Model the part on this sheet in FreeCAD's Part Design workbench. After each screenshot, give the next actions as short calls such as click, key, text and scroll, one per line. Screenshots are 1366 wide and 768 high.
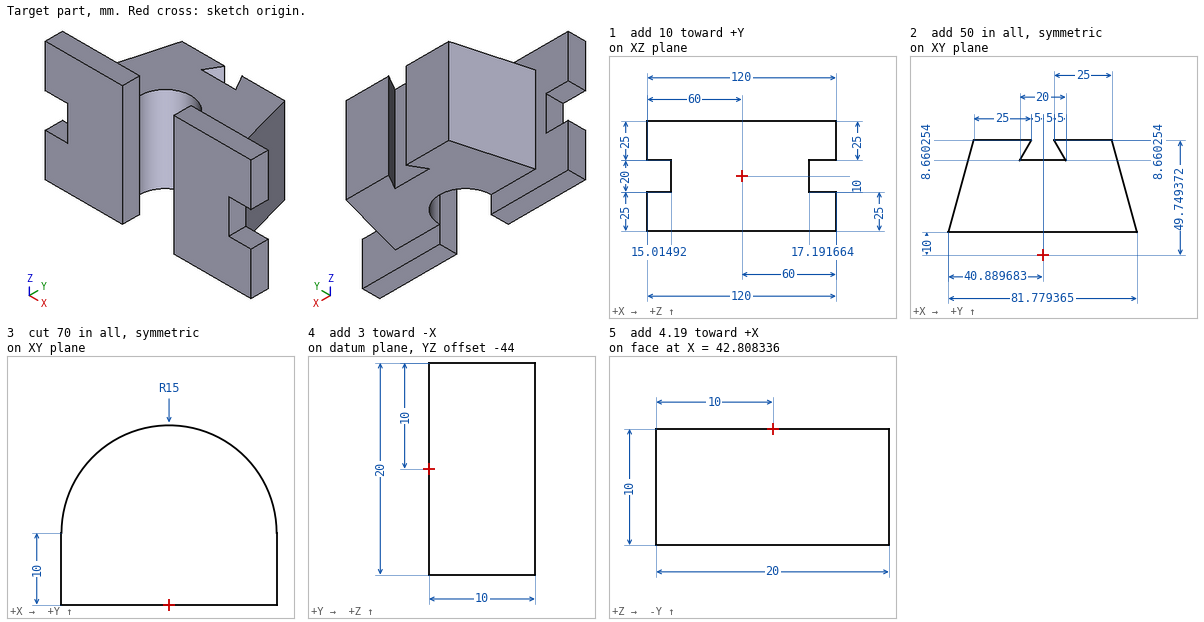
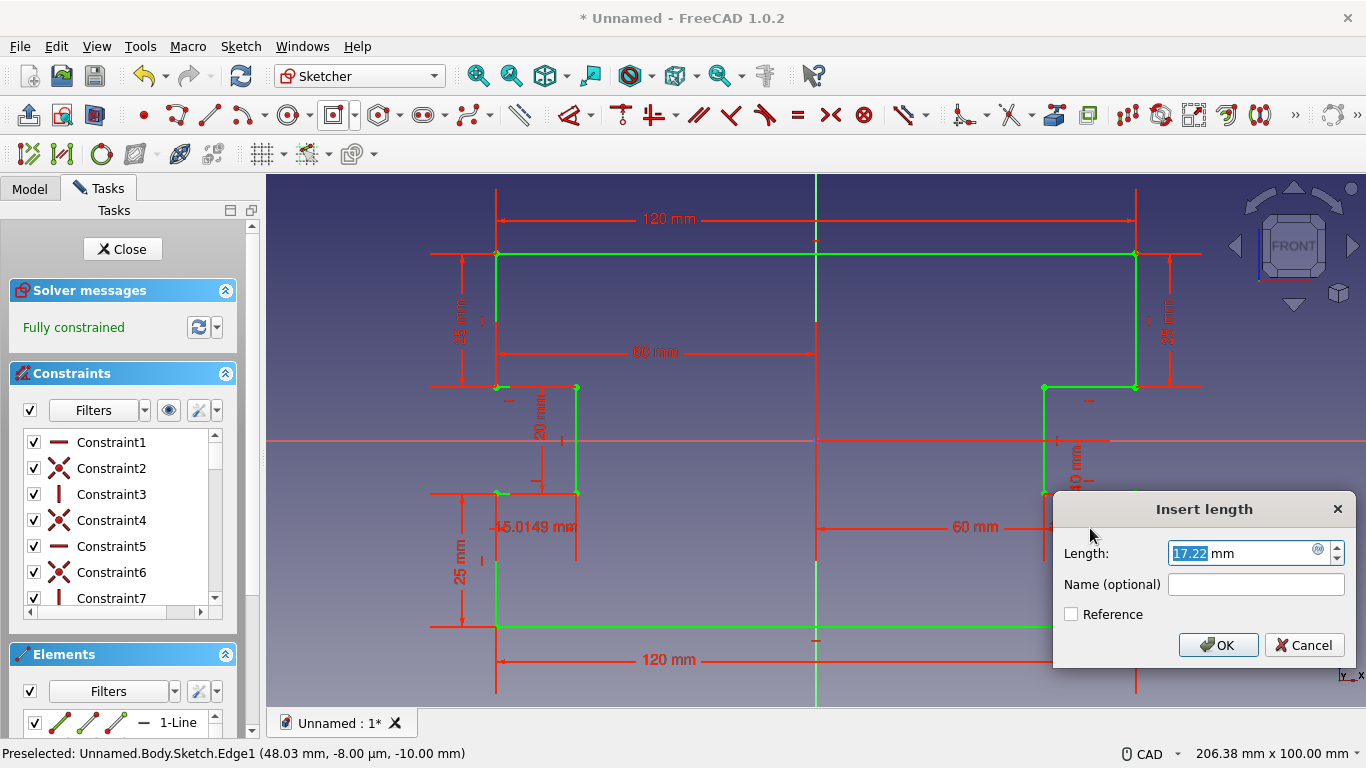
text(17.191664)
key(Return)
key(Escape)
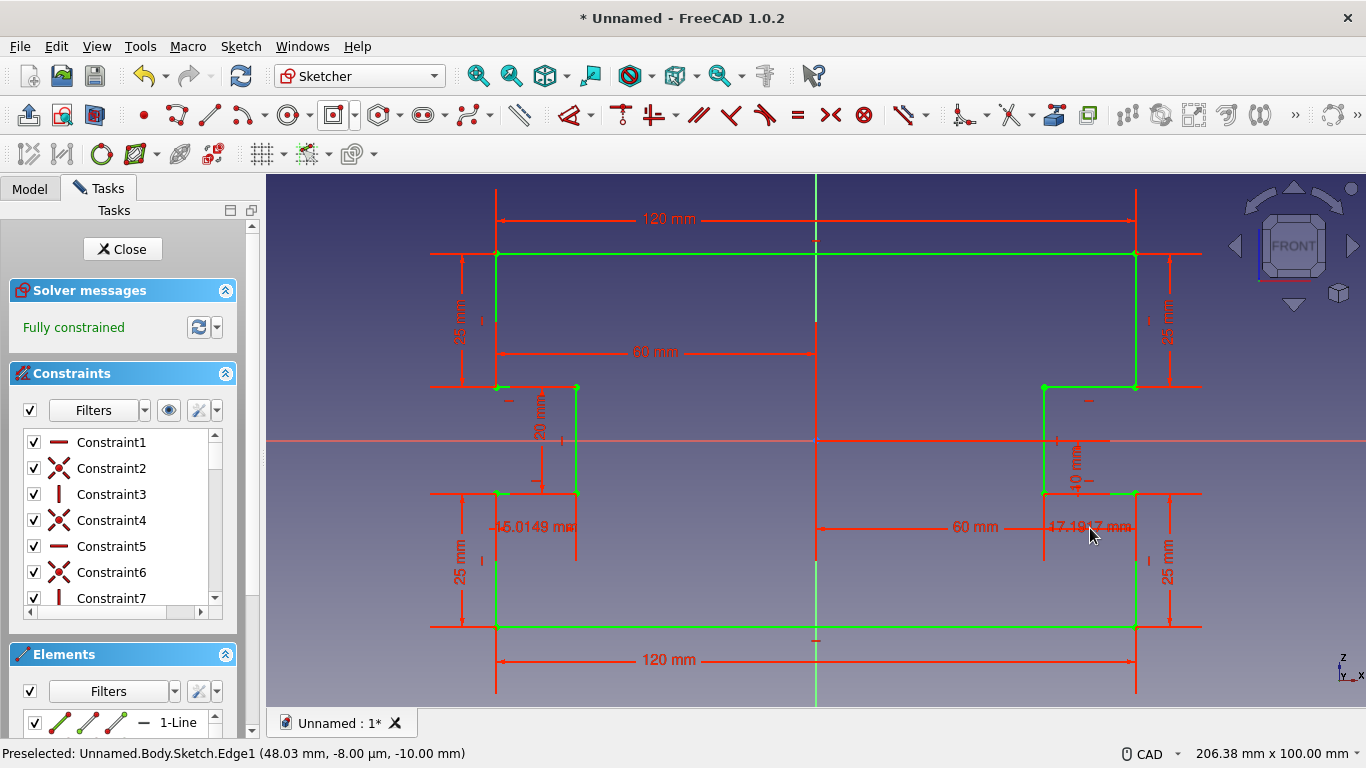
click(123, 249)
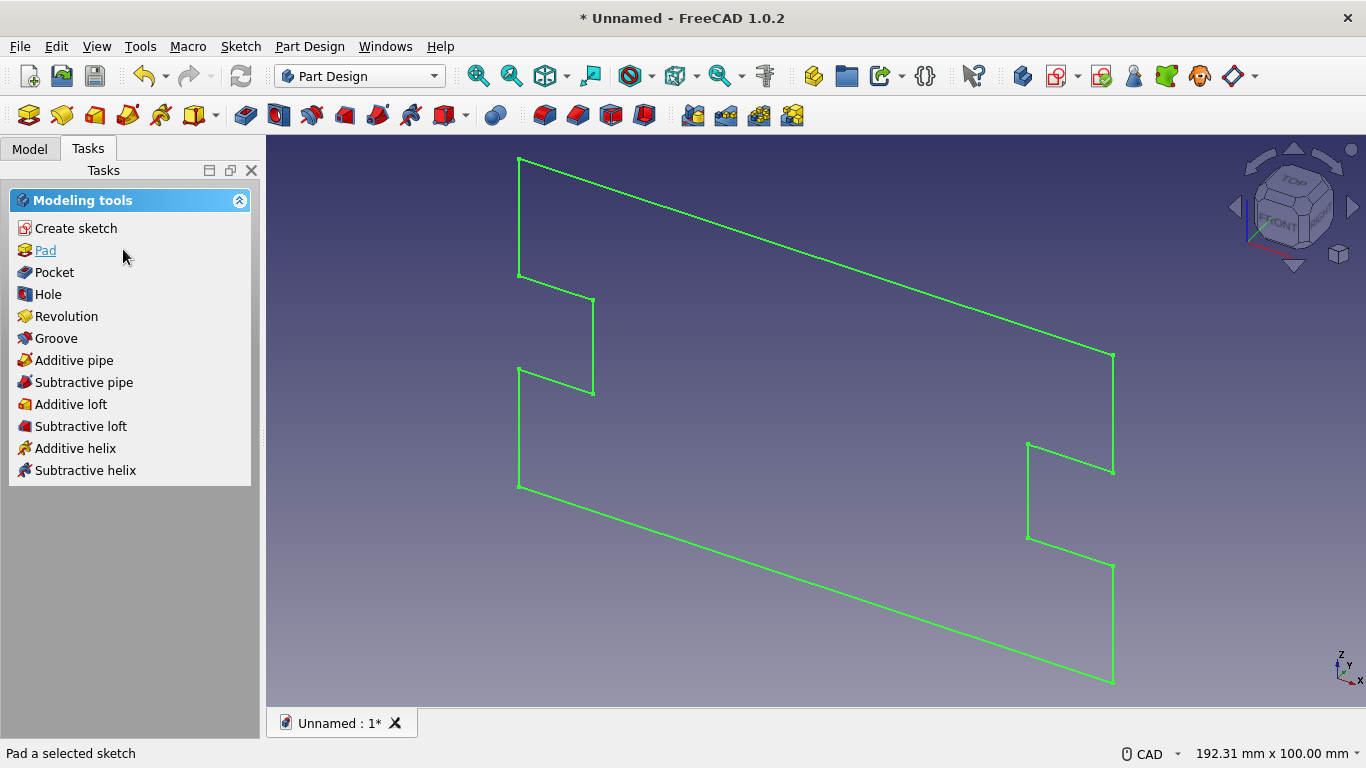
click(29, 116)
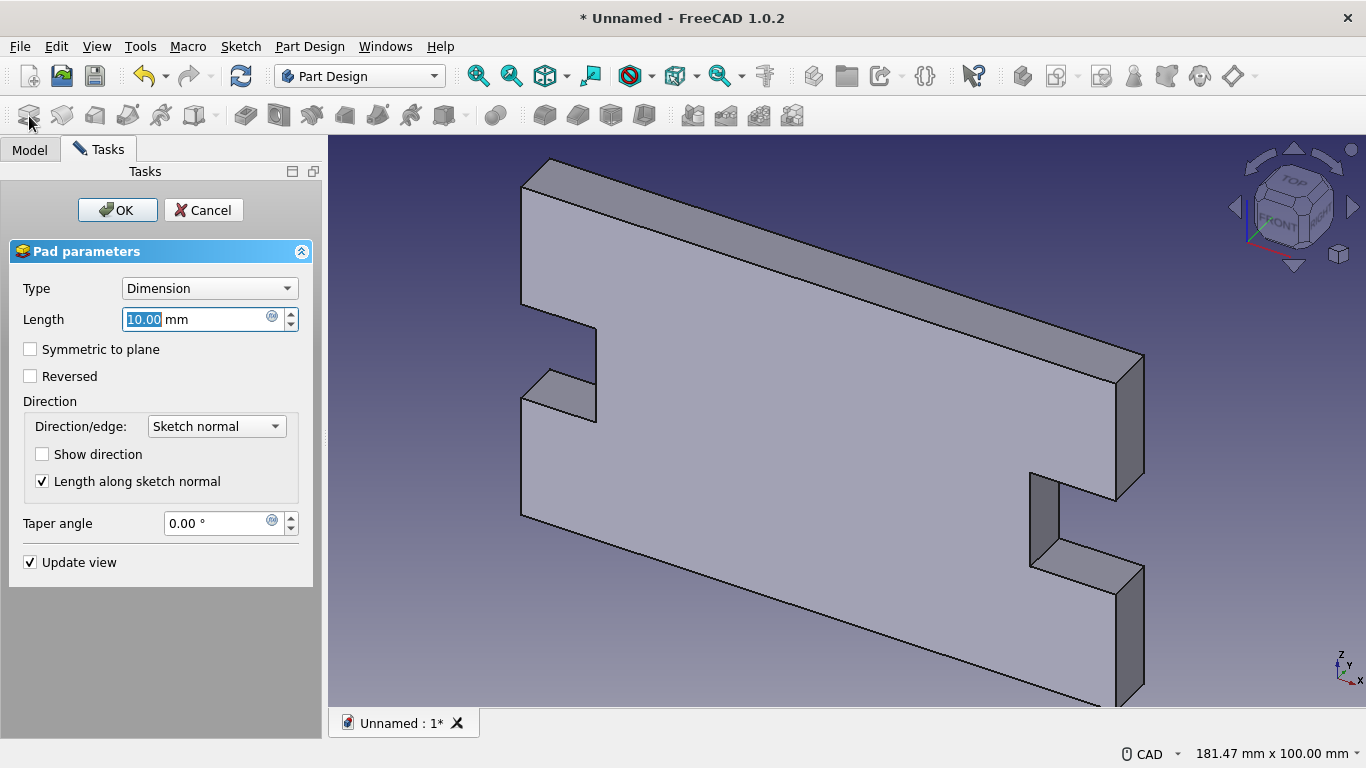
text(10)
key(Tab)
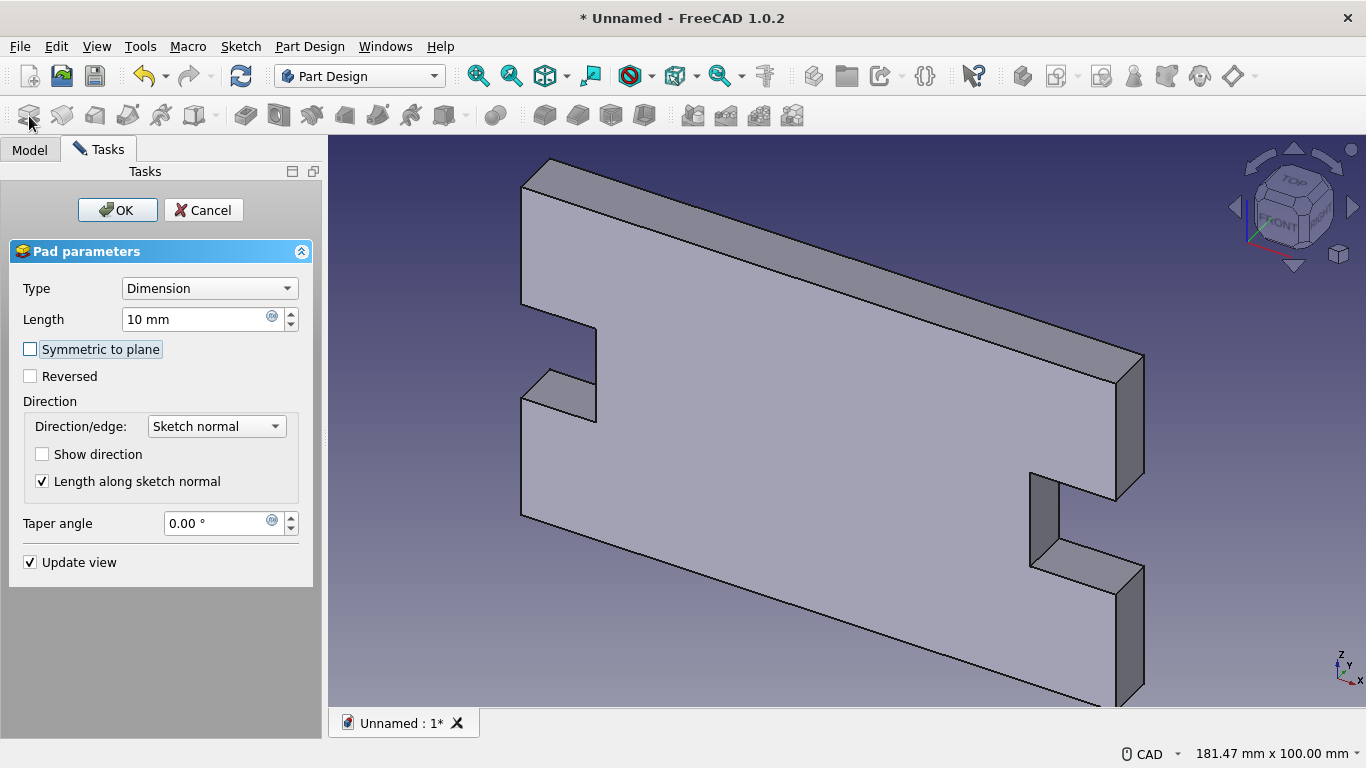
click(31, 376)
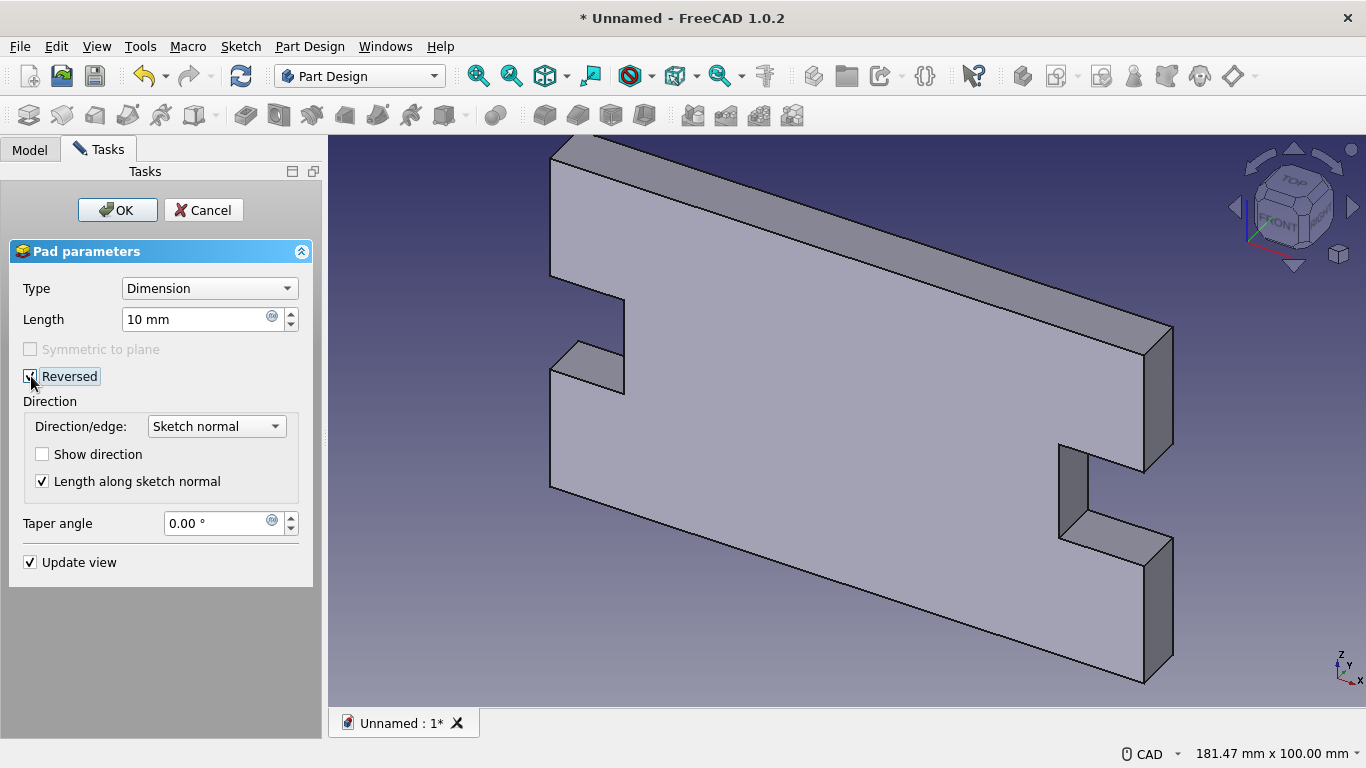
click(118, 210)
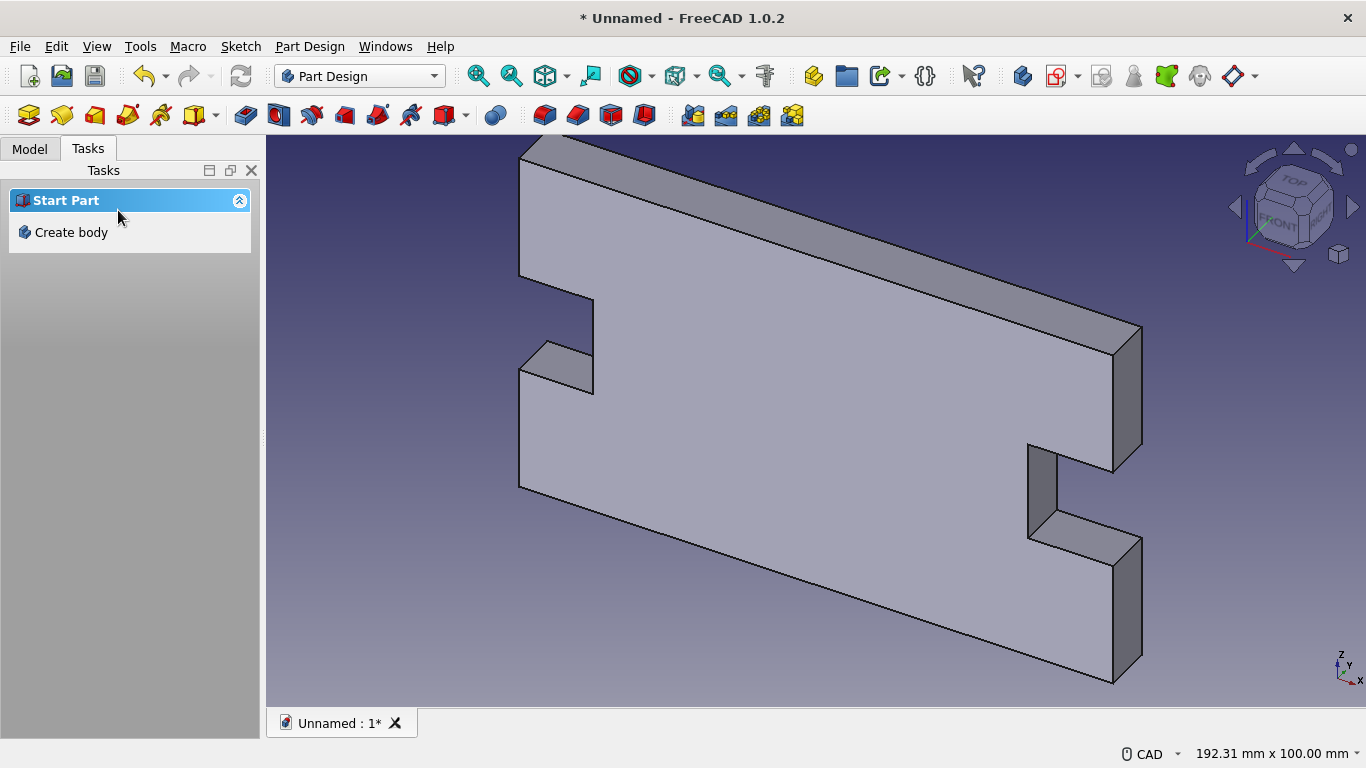
key(v)
key(f)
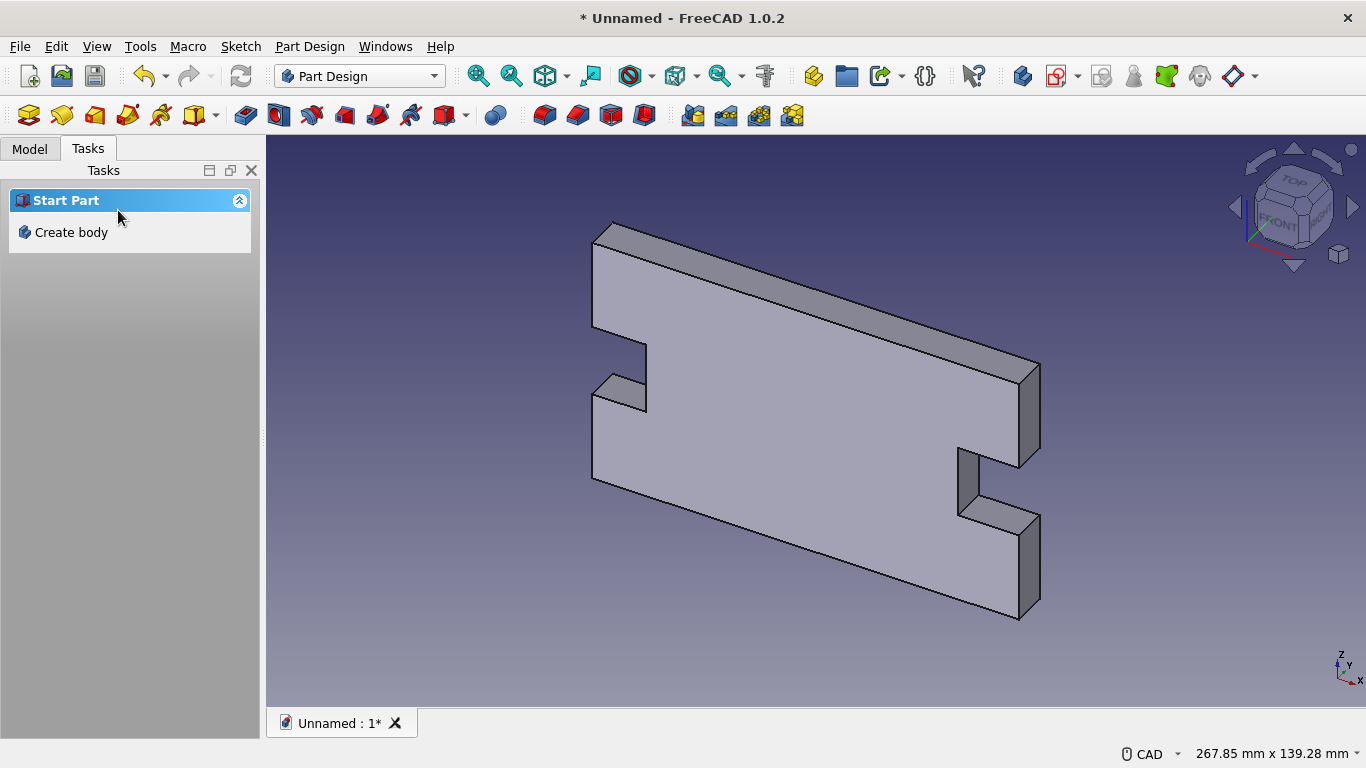
click(1056, 76)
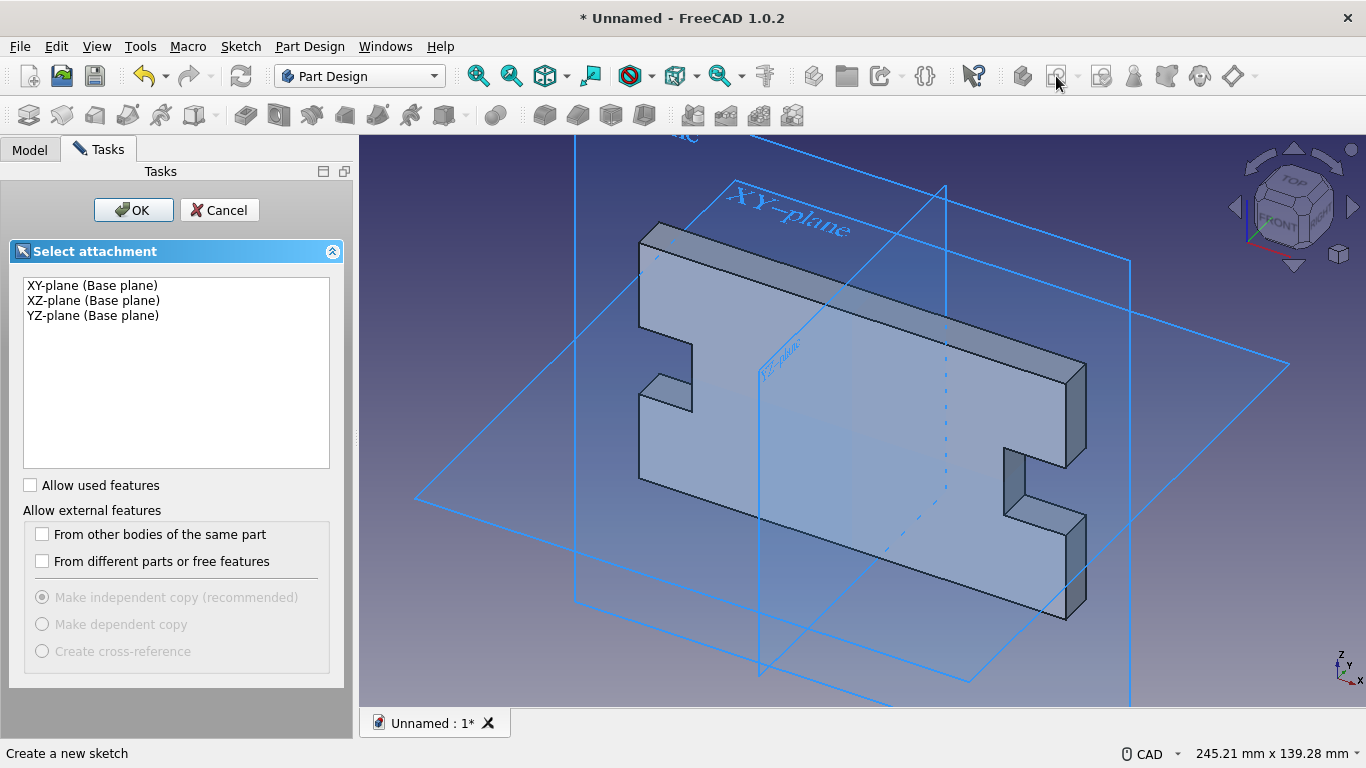
click(84, 286)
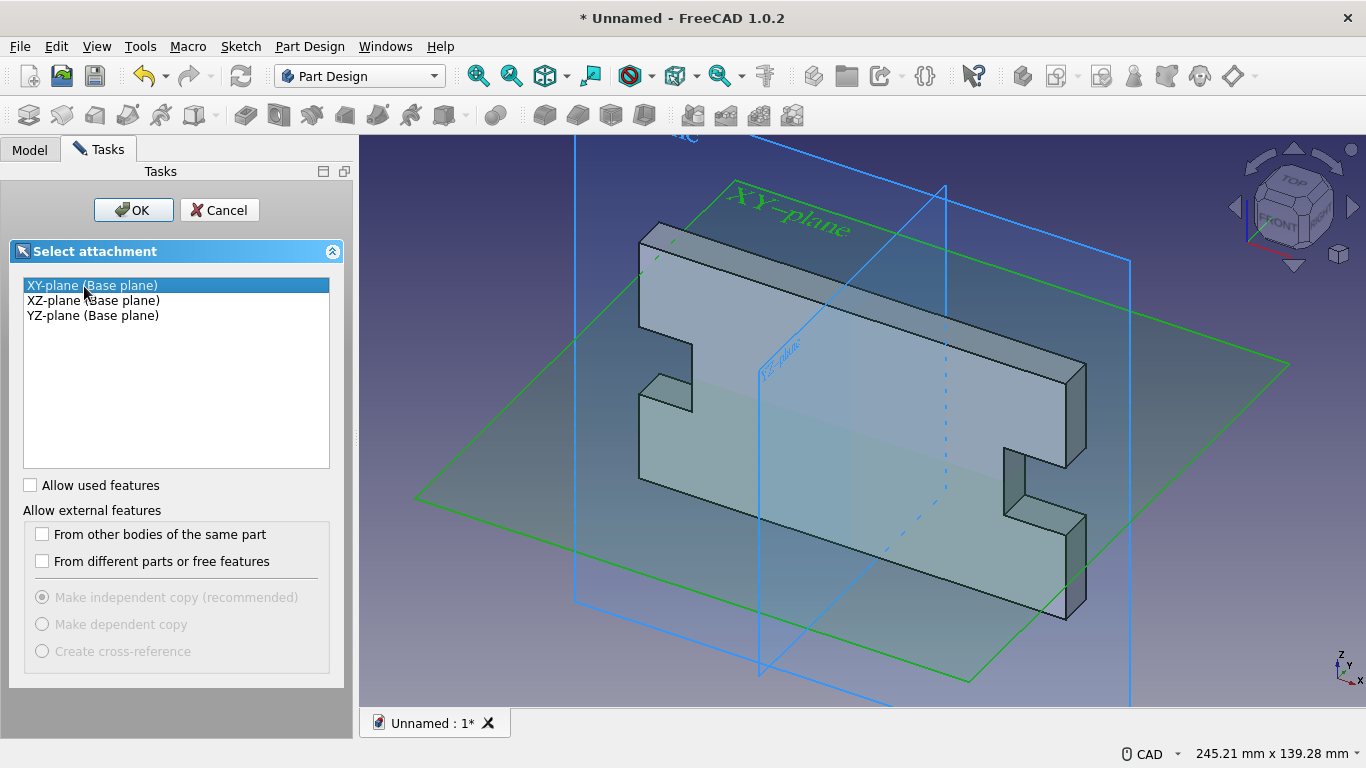
click(134, 210)